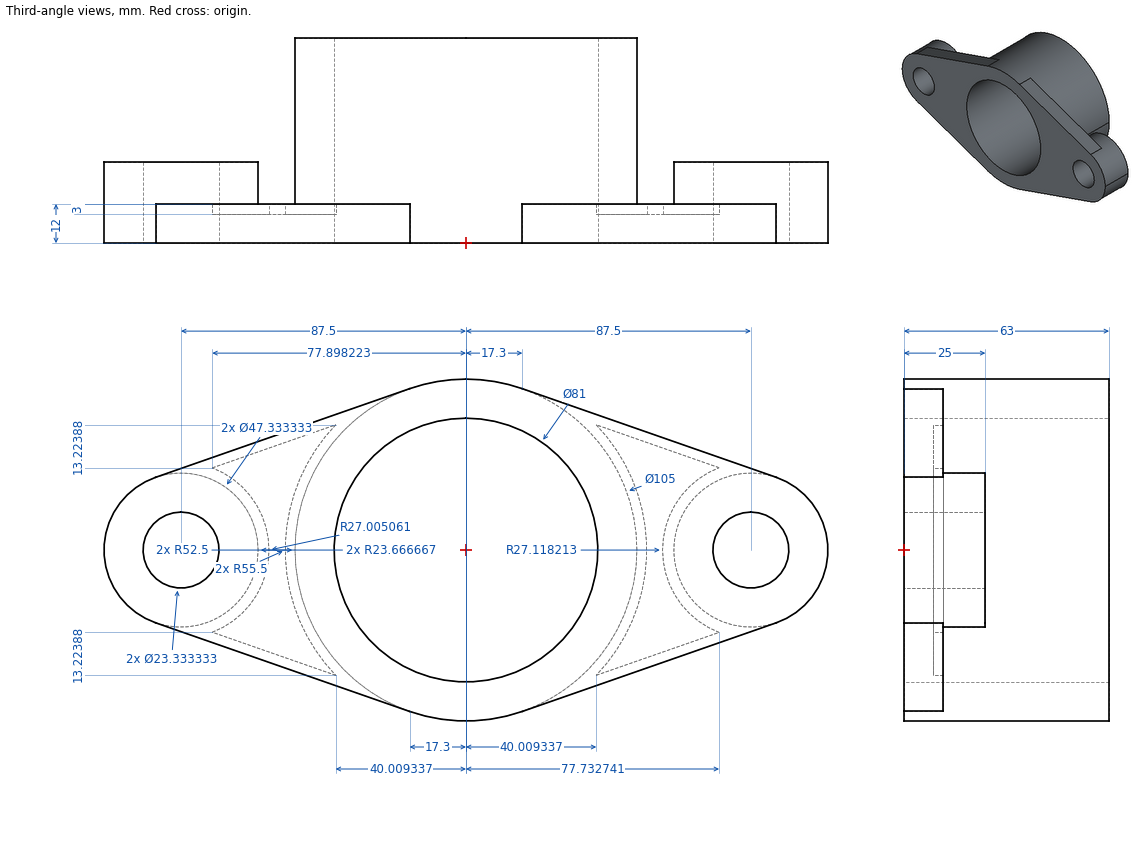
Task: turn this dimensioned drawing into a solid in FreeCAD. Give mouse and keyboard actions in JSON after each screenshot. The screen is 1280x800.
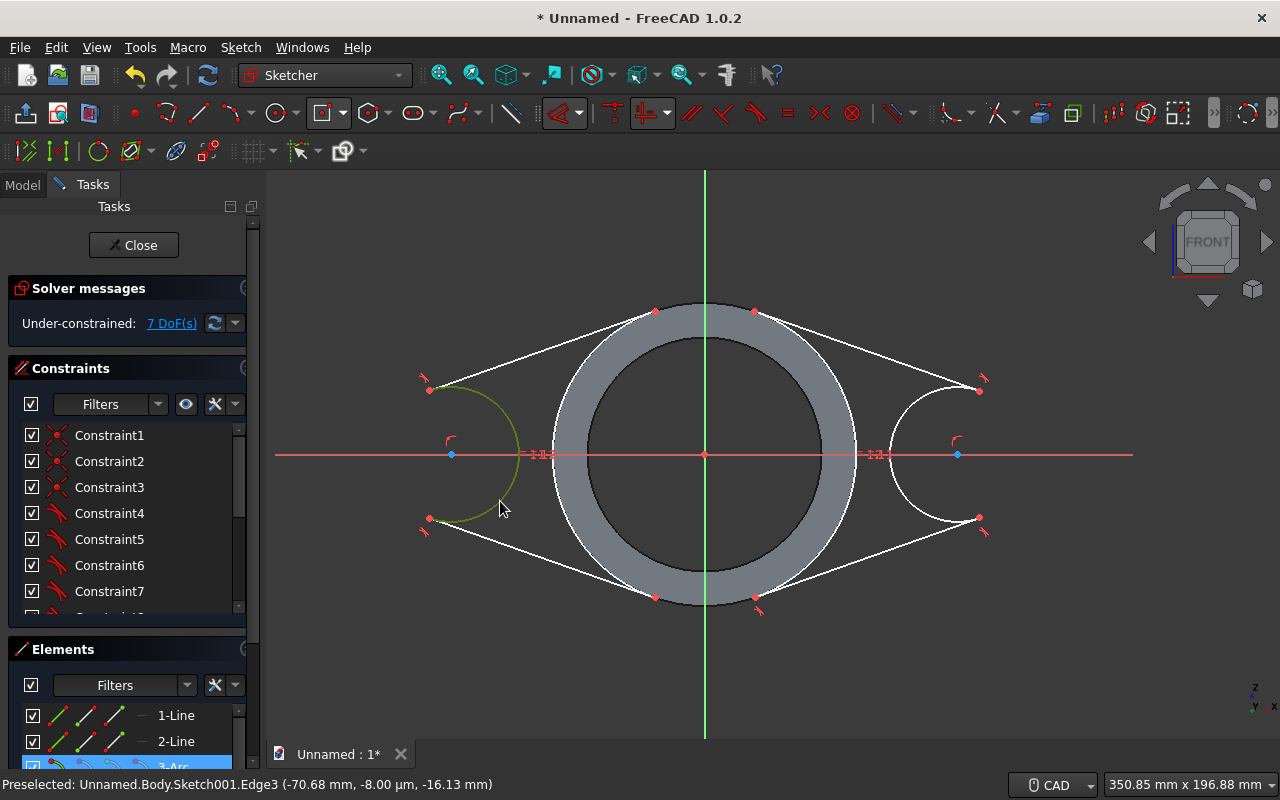
{"action": "key", "text": "k r"}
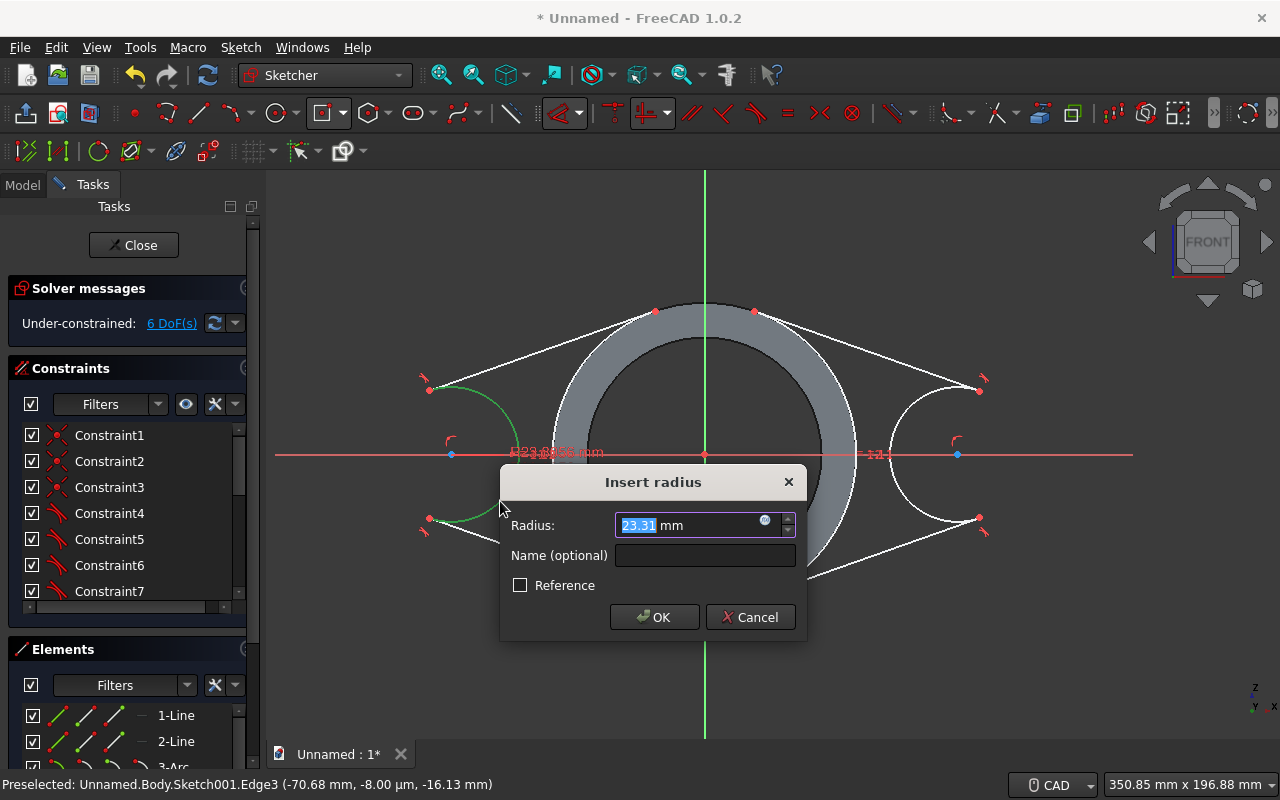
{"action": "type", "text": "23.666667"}
{"action": "key", "text": "Return"}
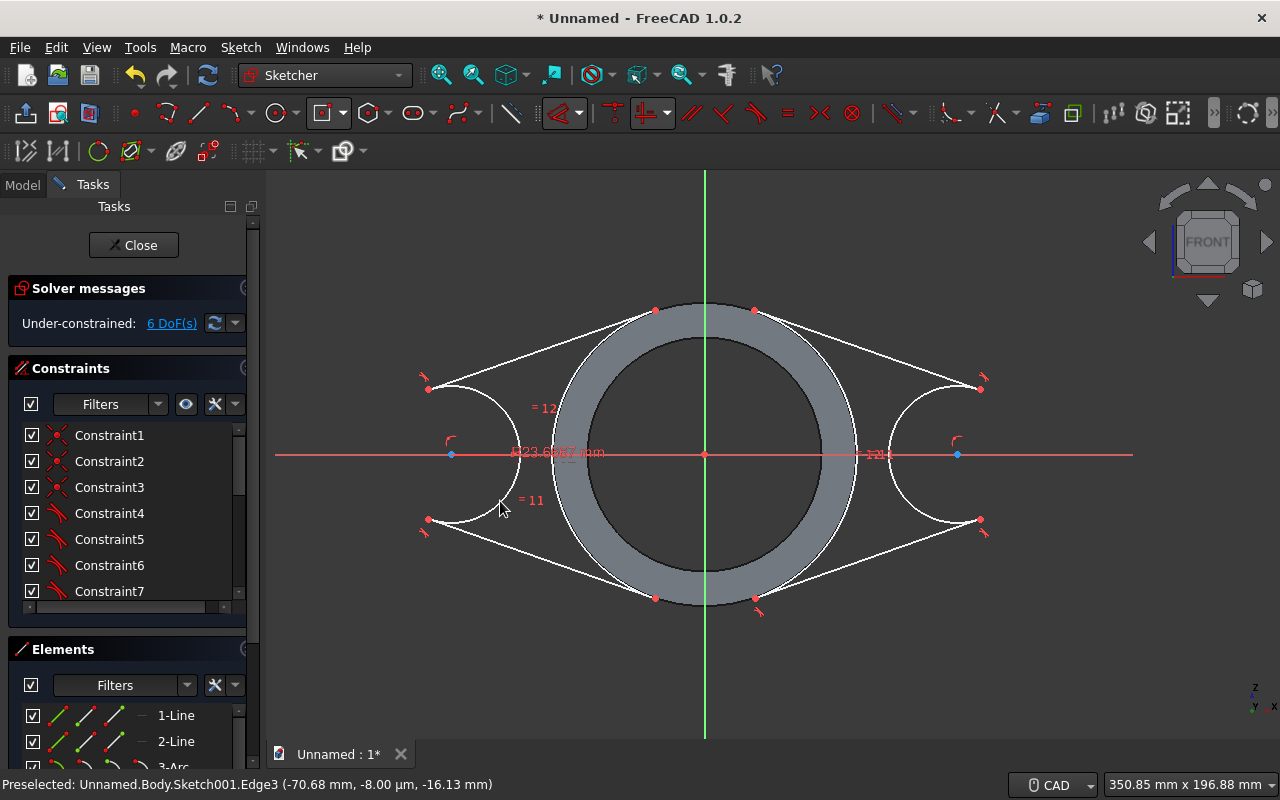
{"action": "left_click", "coordinate": [570, 382]}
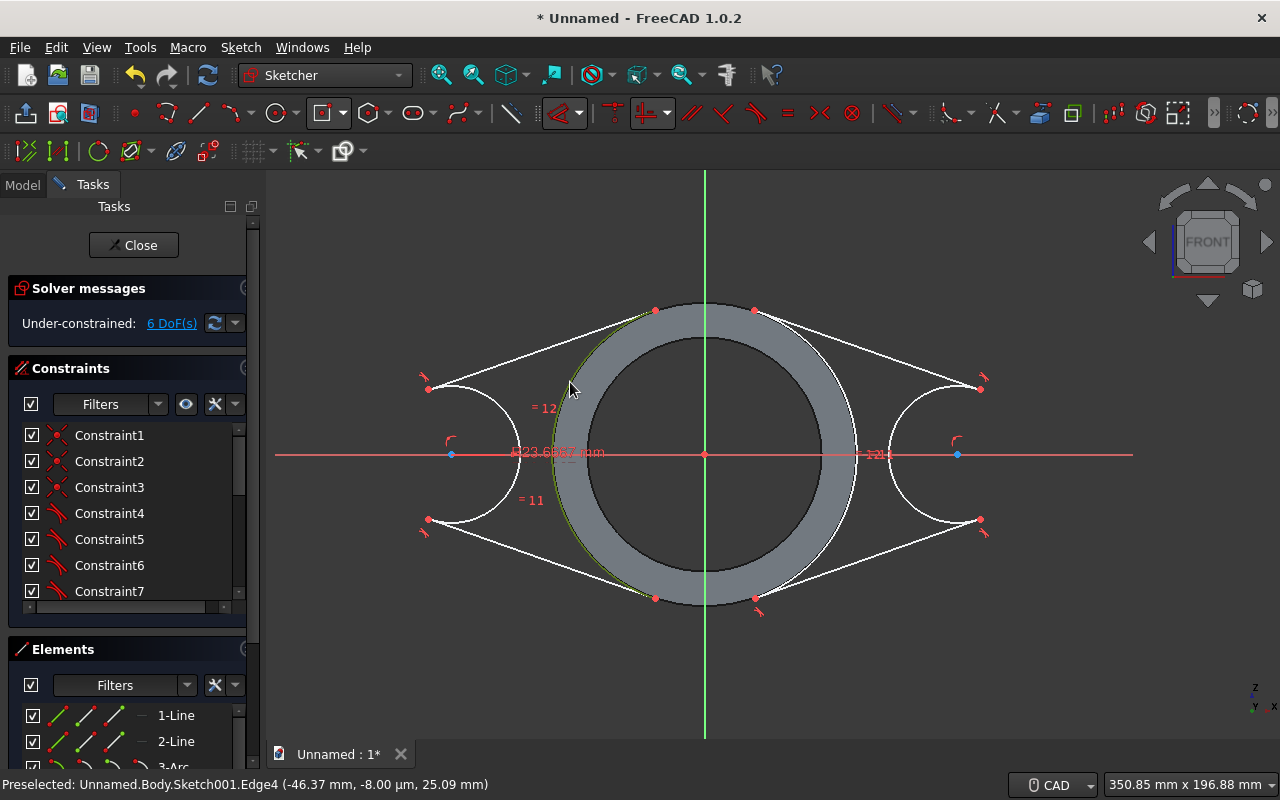
{"action": "key", "text": "k r"}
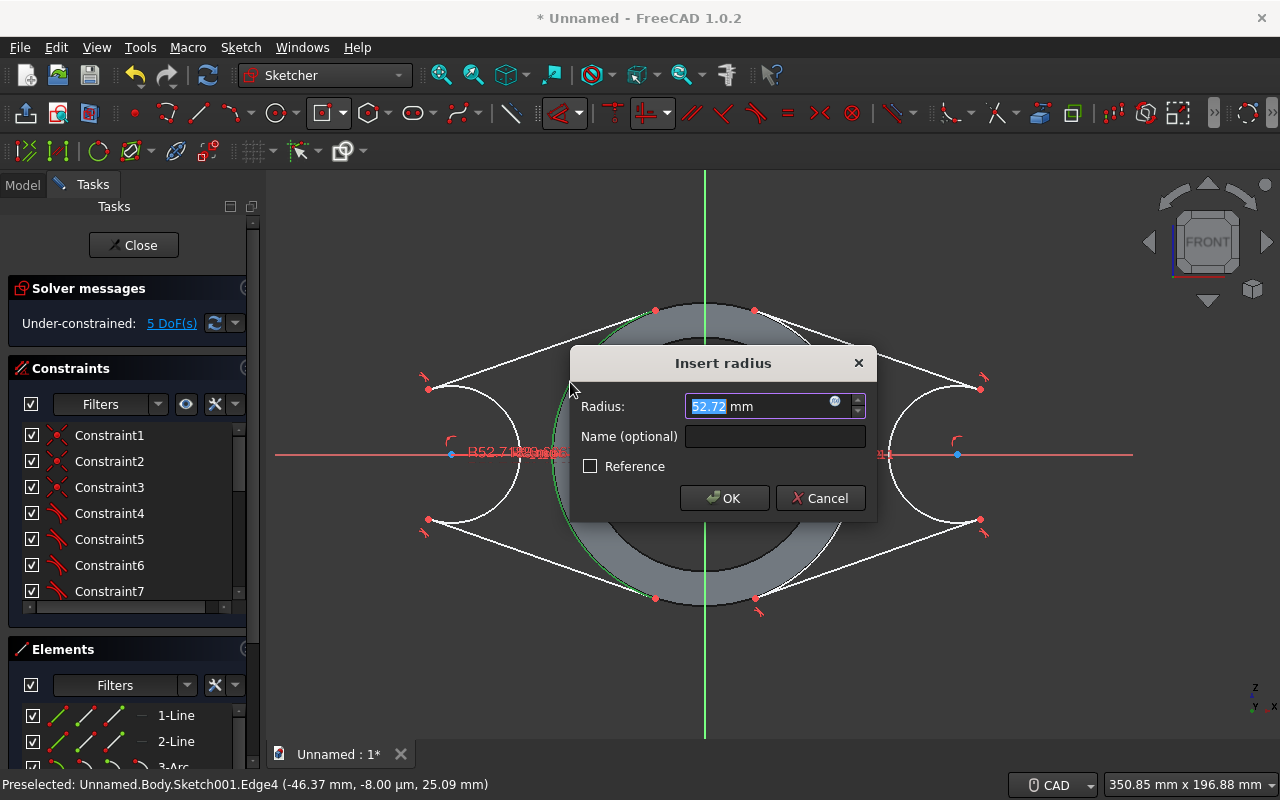
{"action": "type", "text": "52.5"}
{"action": "key", "text": "Return"}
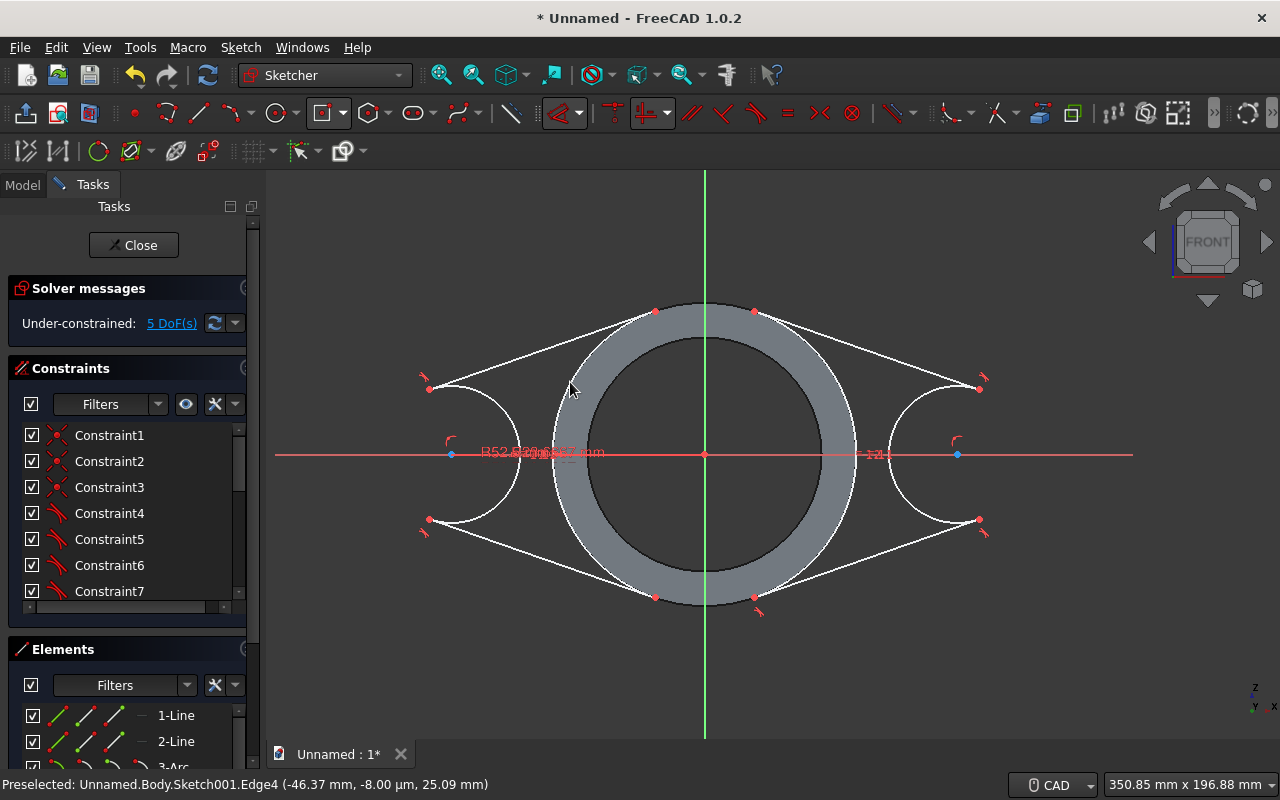
{"action": "left_click", "coordinate": [655, 598]}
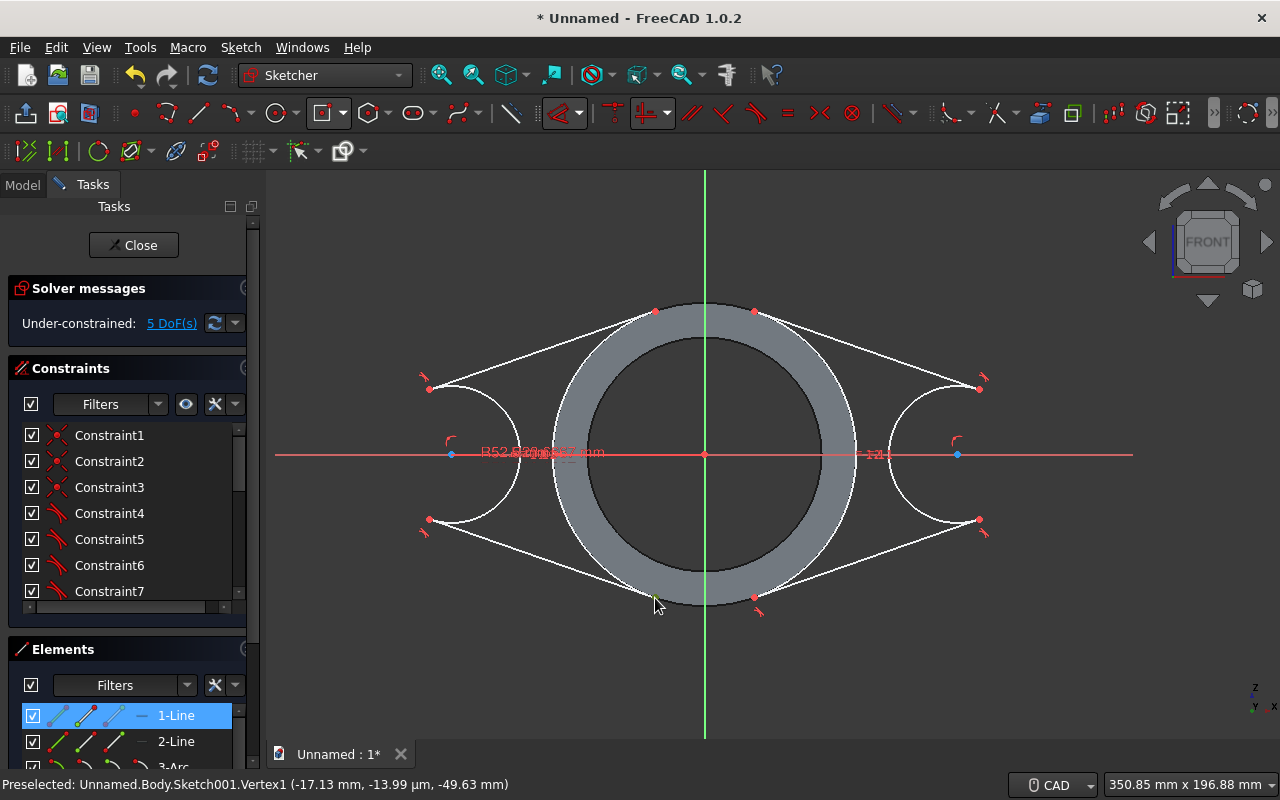
{"action": "key", "text": "l"}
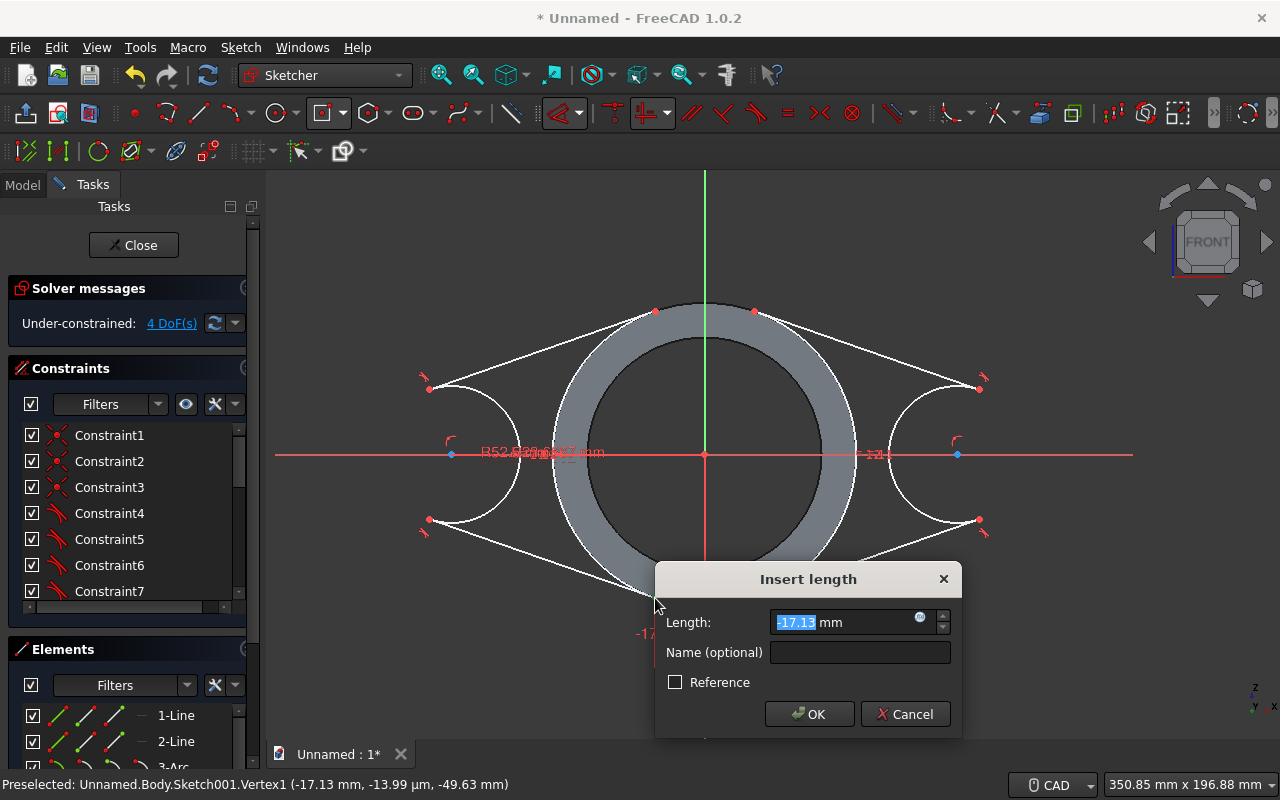
{"action": "type", "text": "-17.3"}
{"action": "key", "text": "Return"}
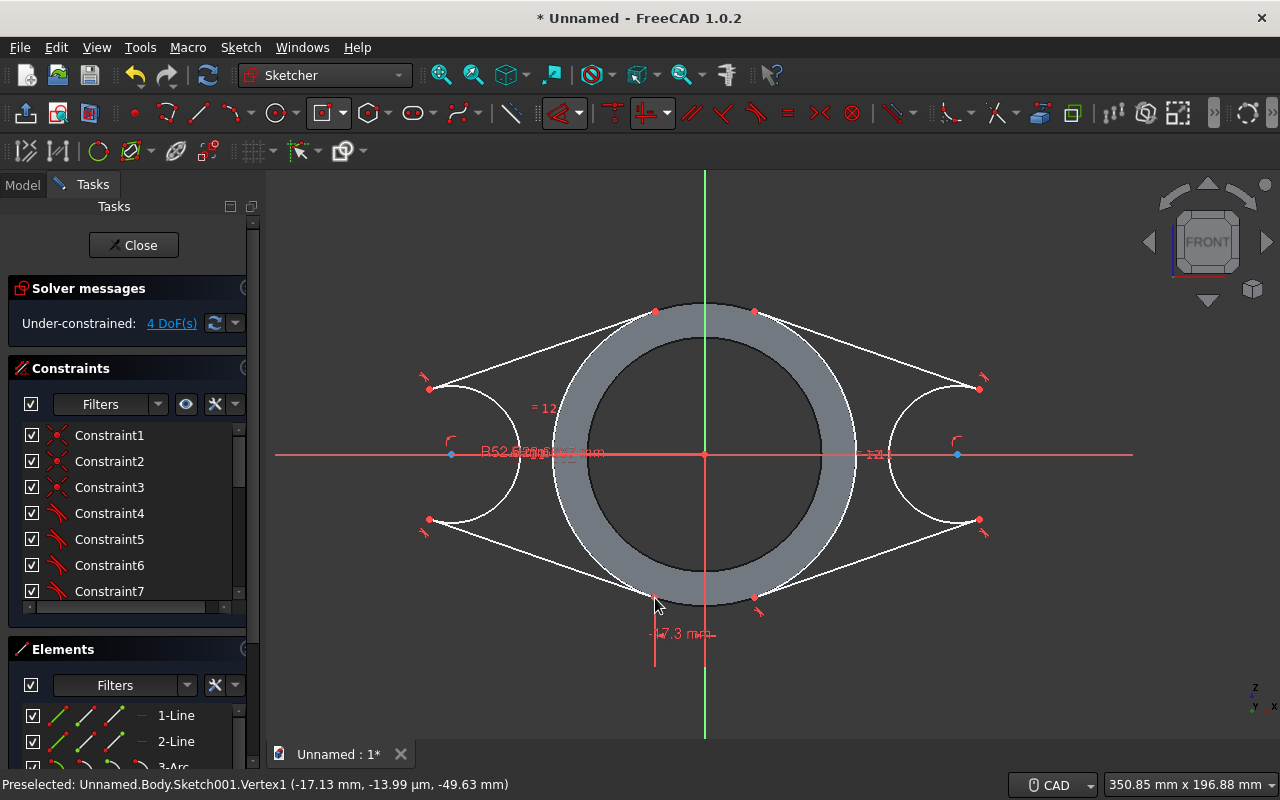
{"action": "left_click", "coordinate": [655, 311]}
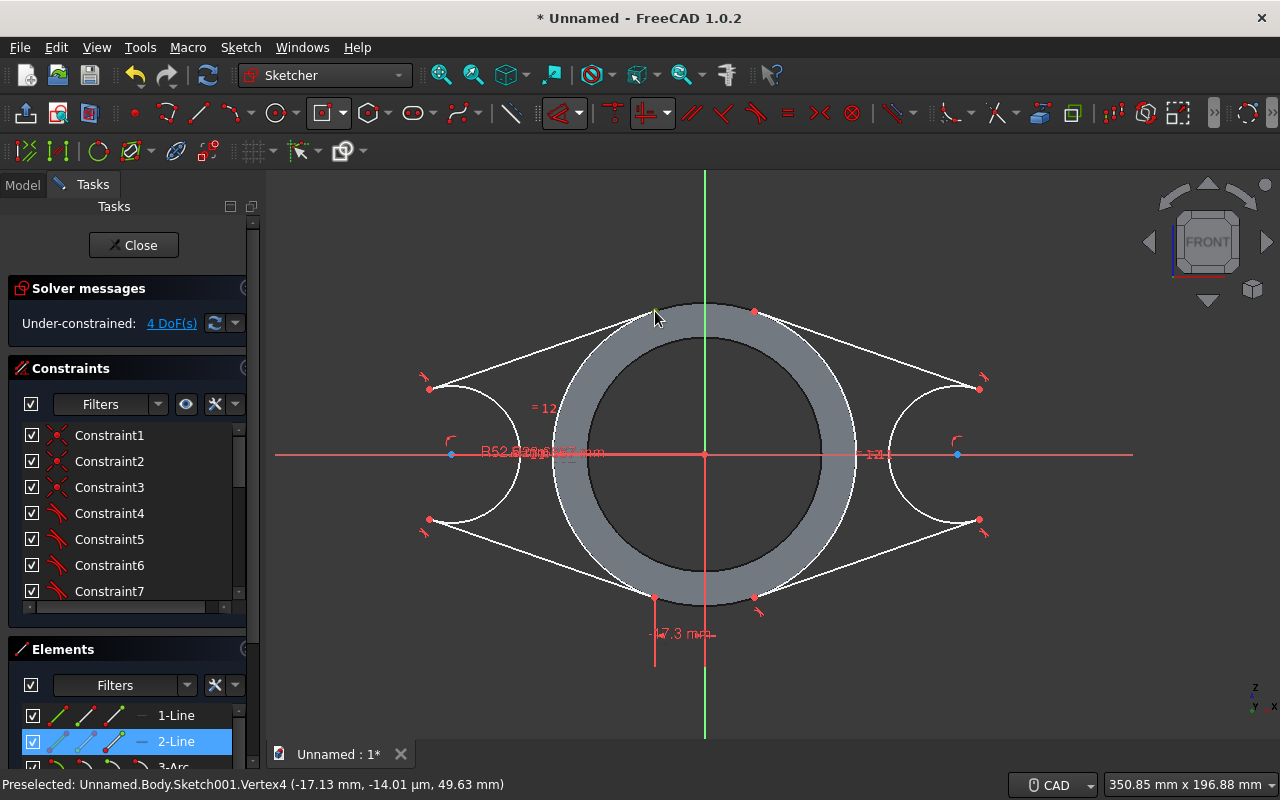
{"action": "left_click", "coordinate": [582, 114]}